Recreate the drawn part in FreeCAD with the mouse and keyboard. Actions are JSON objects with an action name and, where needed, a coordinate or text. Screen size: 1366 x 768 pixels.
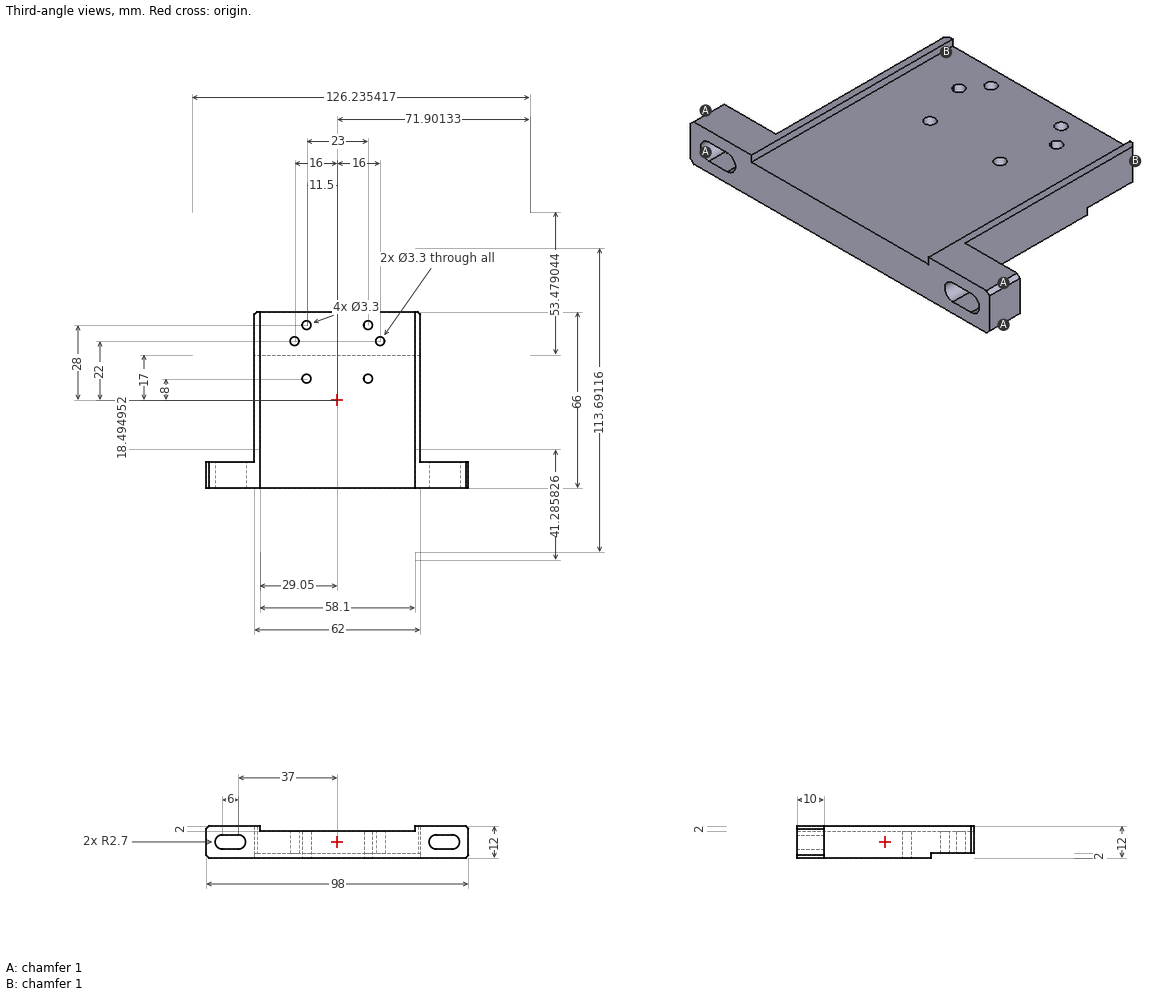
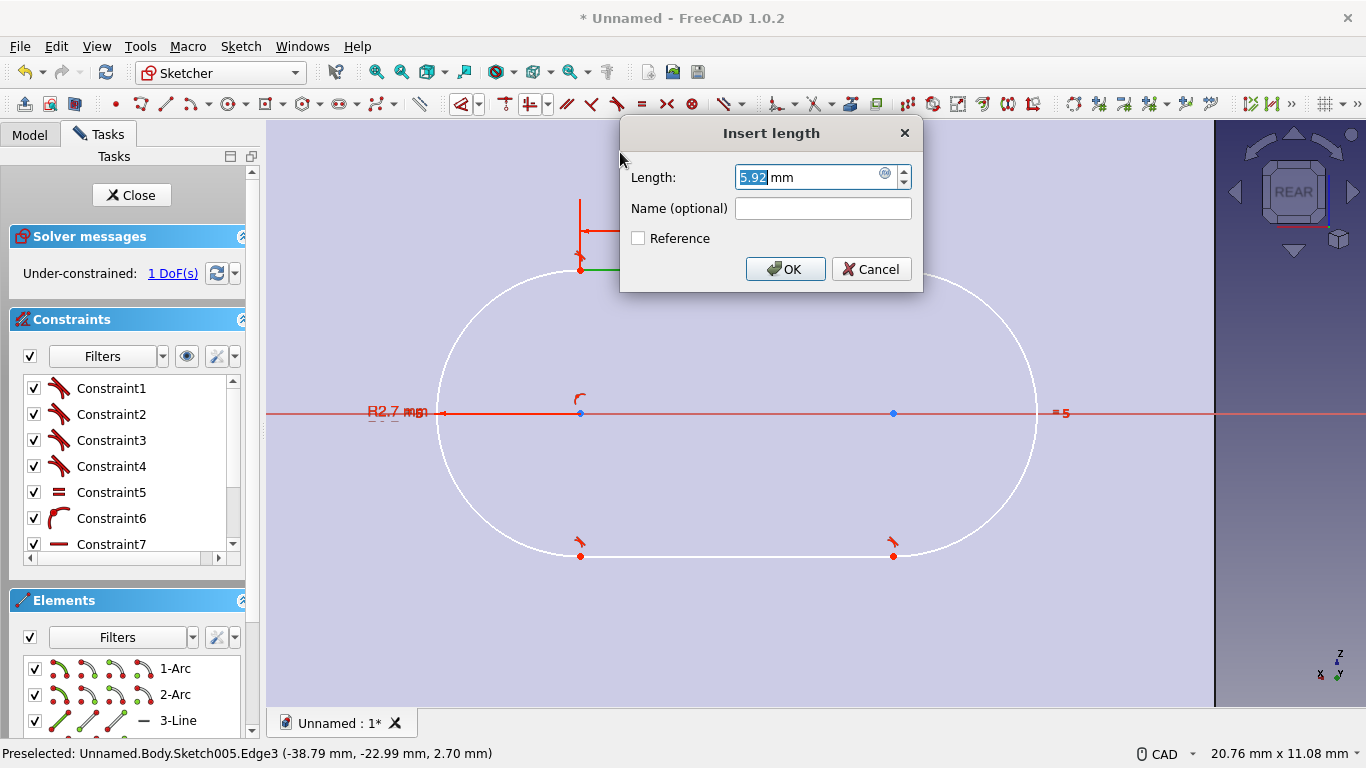
{"action": "type", "text": "6"}
{"action": "key", "text": "Return"}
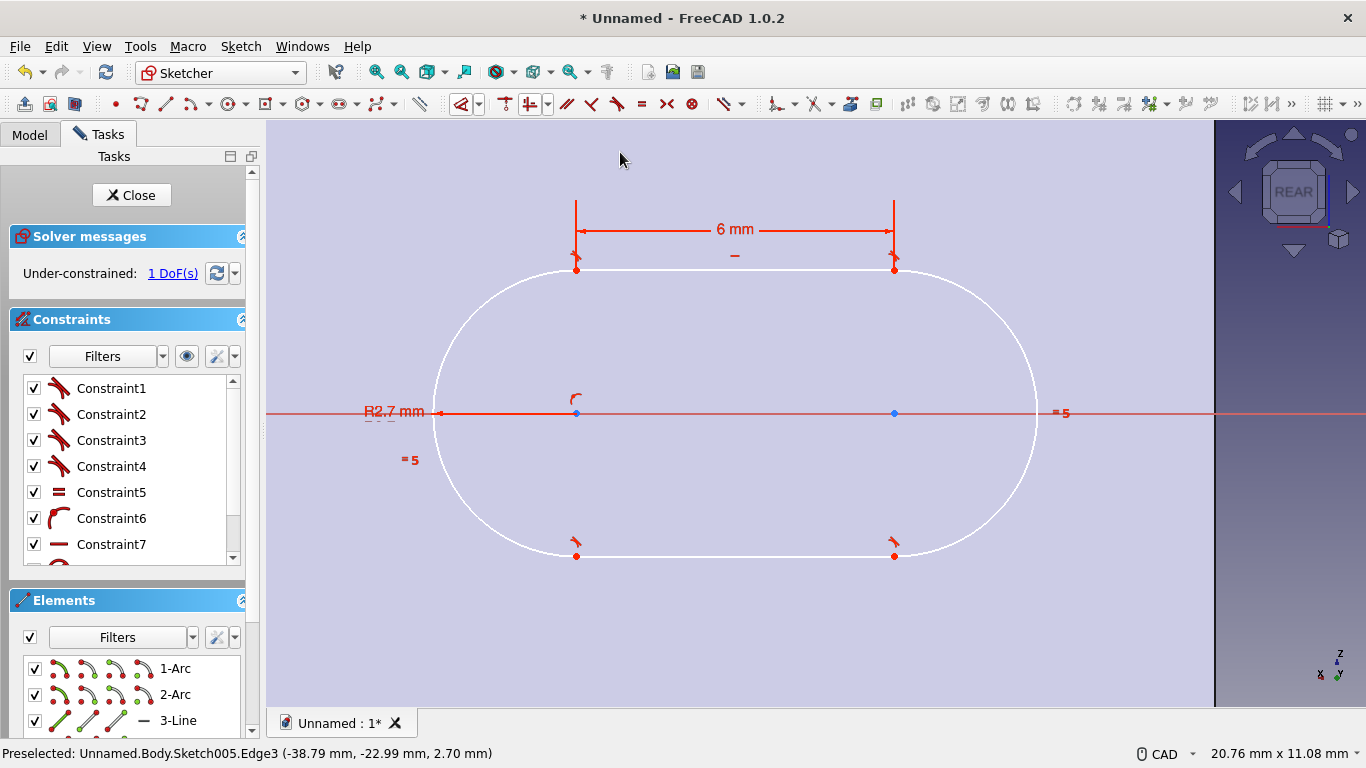
{"action": "left_click", "coordinate": [576, 270]}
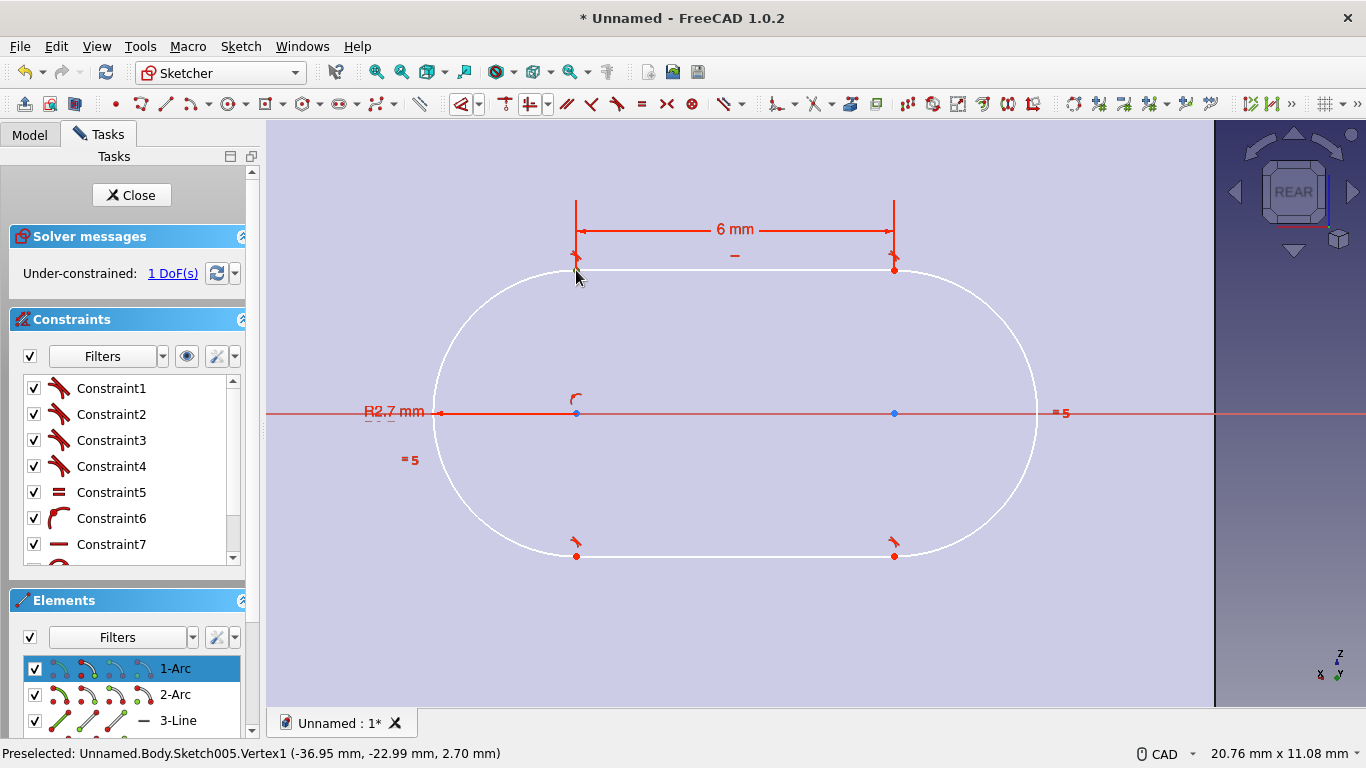
{"action": "left_click", "coordinate": [478, 104]}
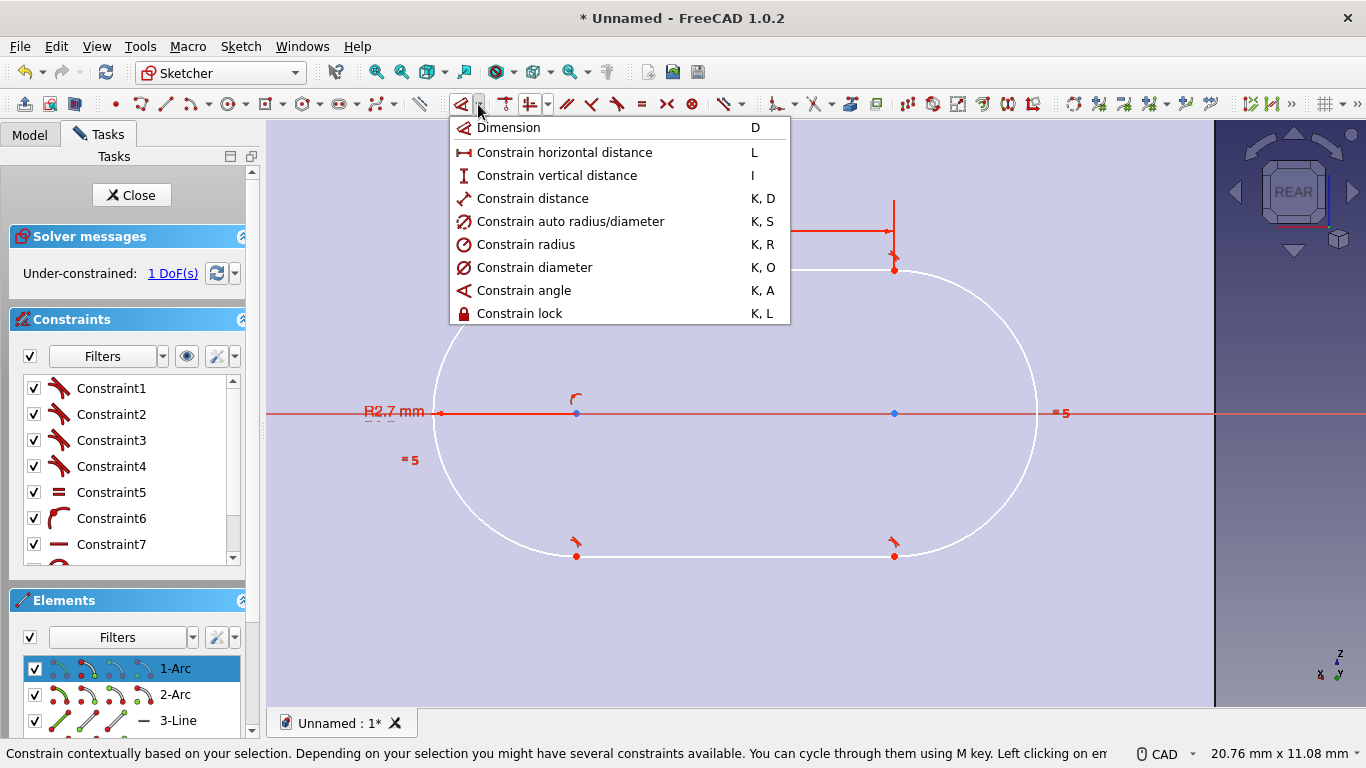
{"action": "left_click", "coordinate": [620, 152]}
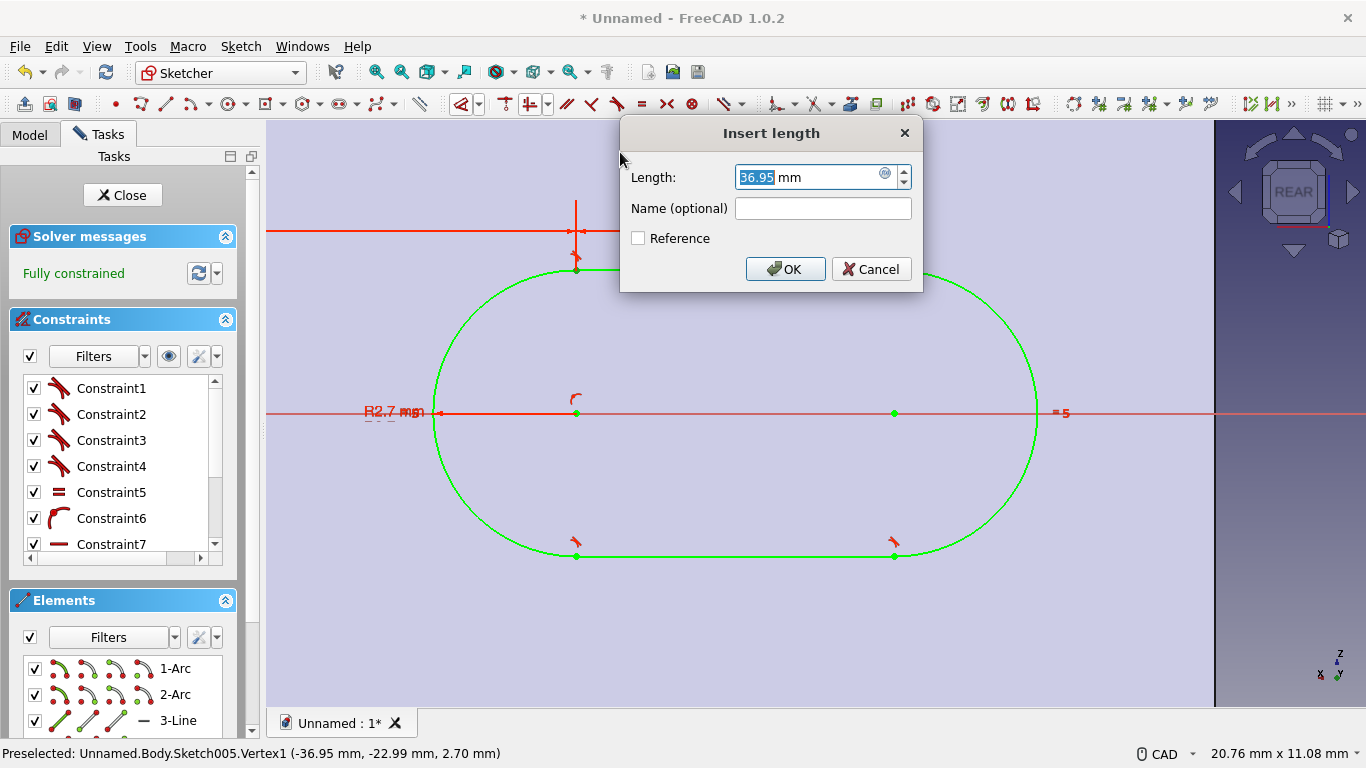
{"action": "type", "text": "37"}
{"action": "key", "text": "Return"}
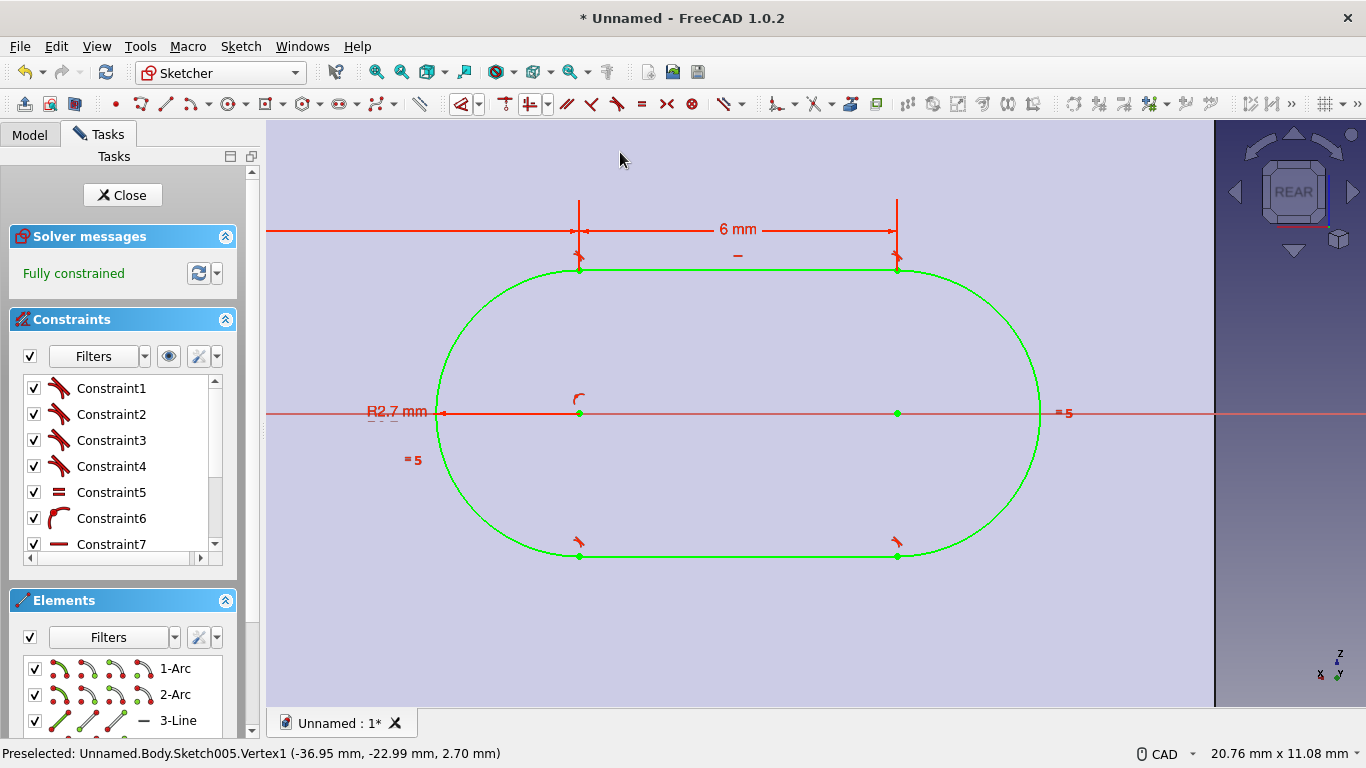
{"action": "left_click", "coordinate": [123, 195]}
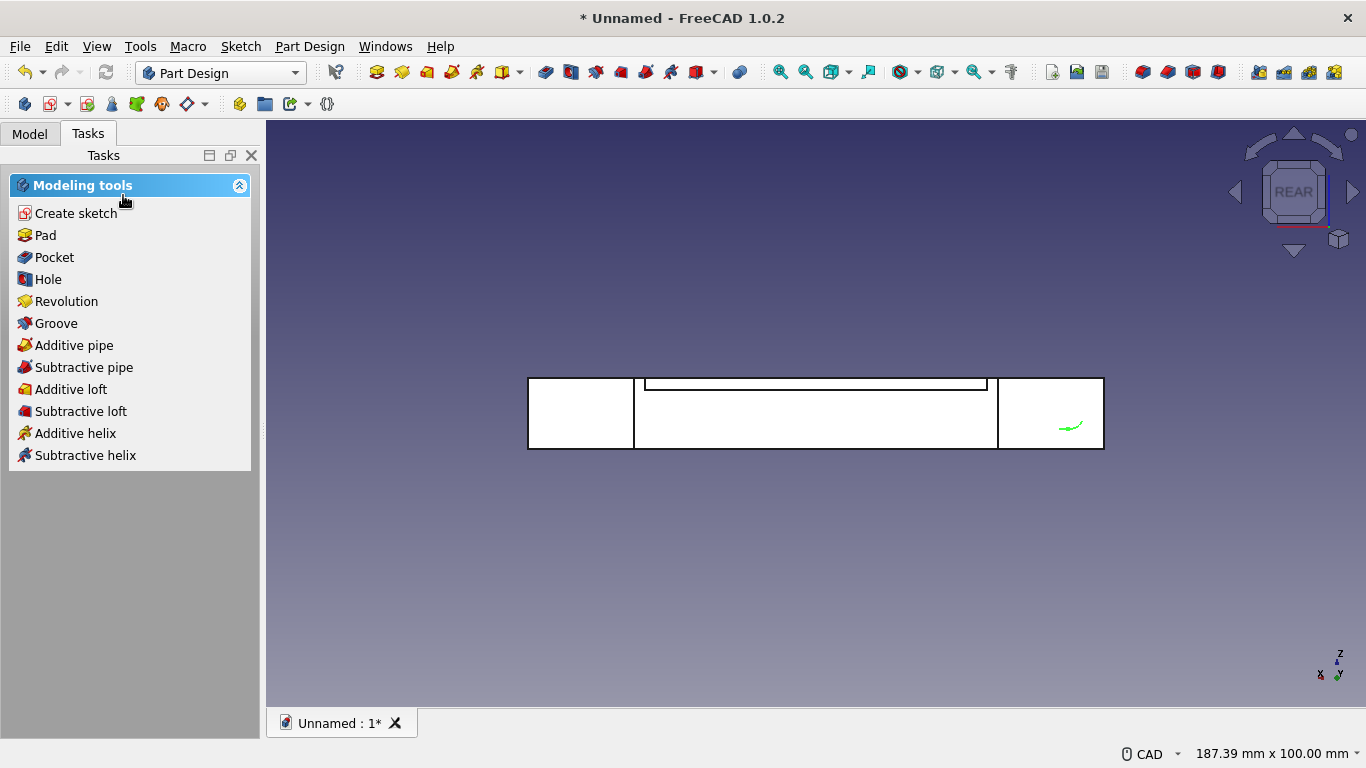
{"action": "left_click", "coordinate": [546, 72]}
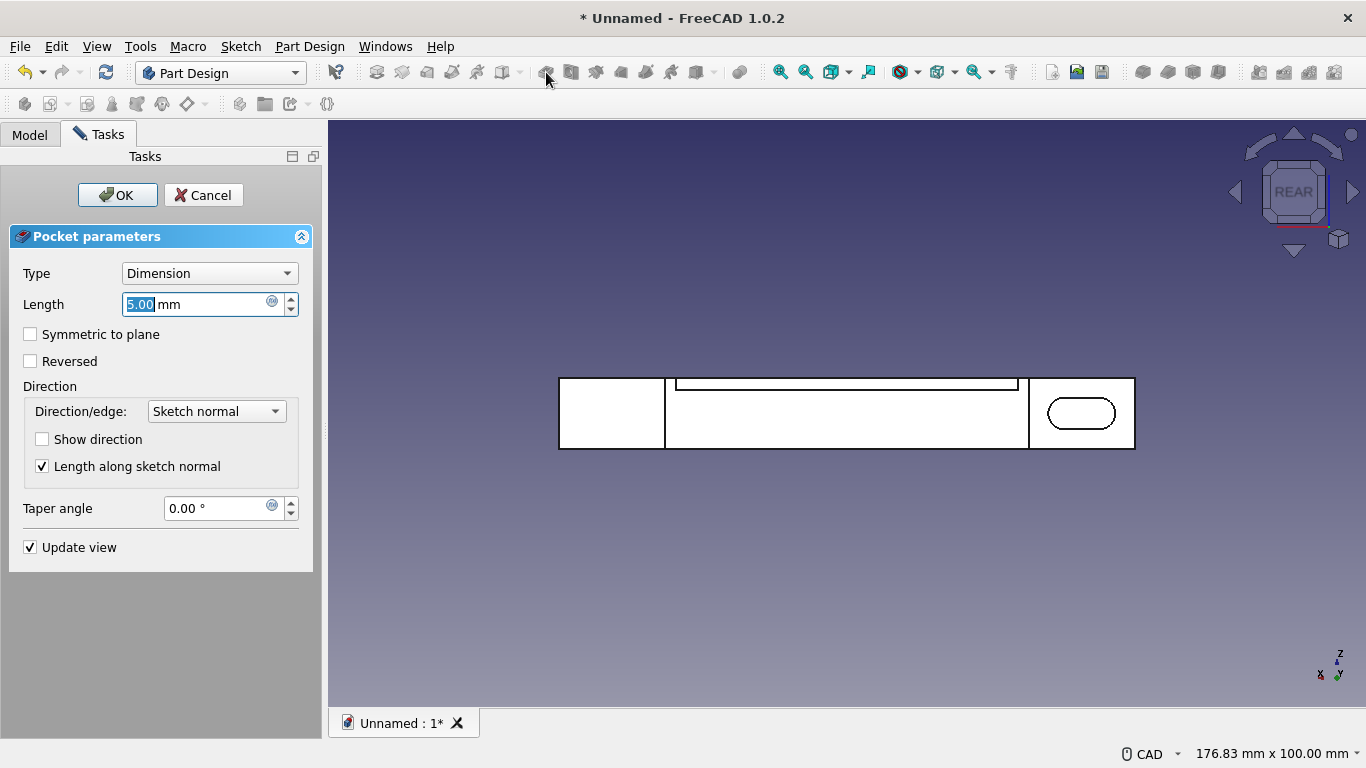
{"action": "left_click", "coordinate": [210, 274]}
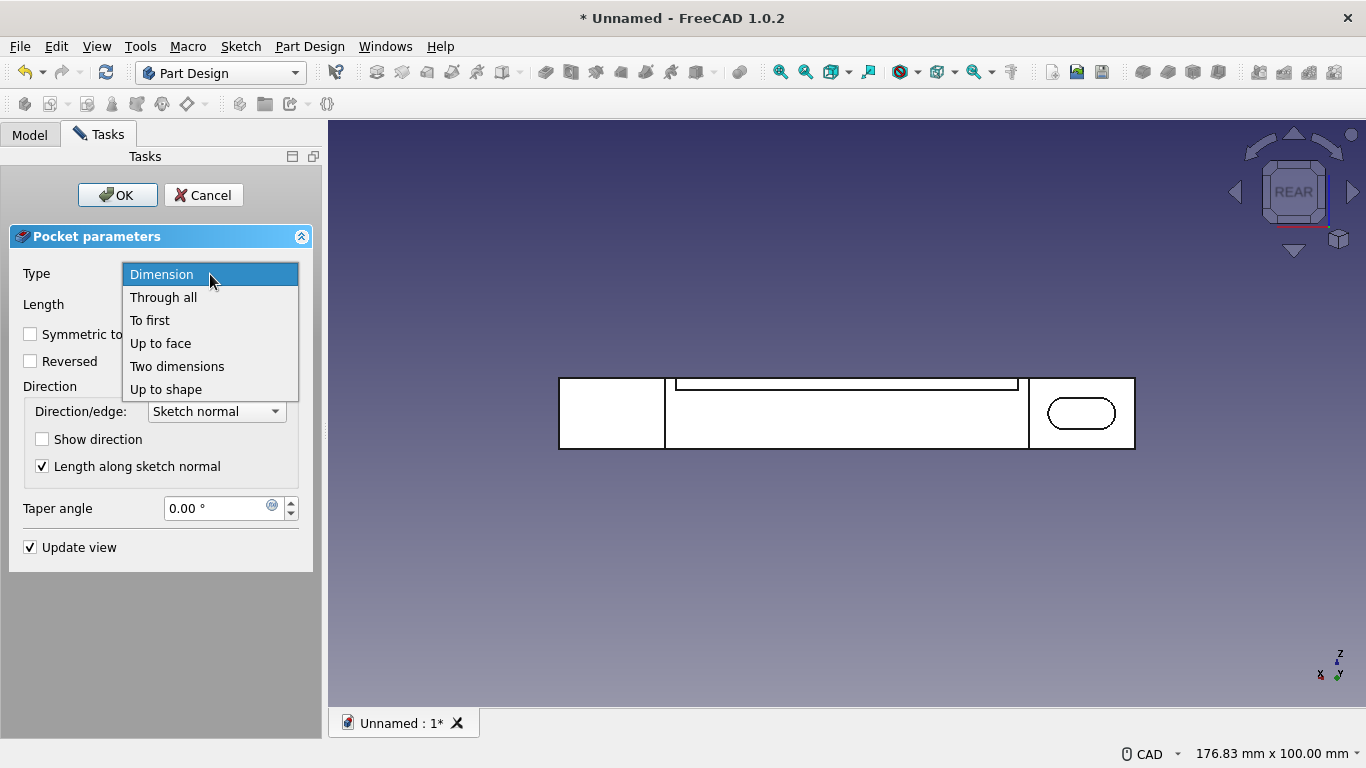
{"action": "left_click", "coordinate": [208, 298]}